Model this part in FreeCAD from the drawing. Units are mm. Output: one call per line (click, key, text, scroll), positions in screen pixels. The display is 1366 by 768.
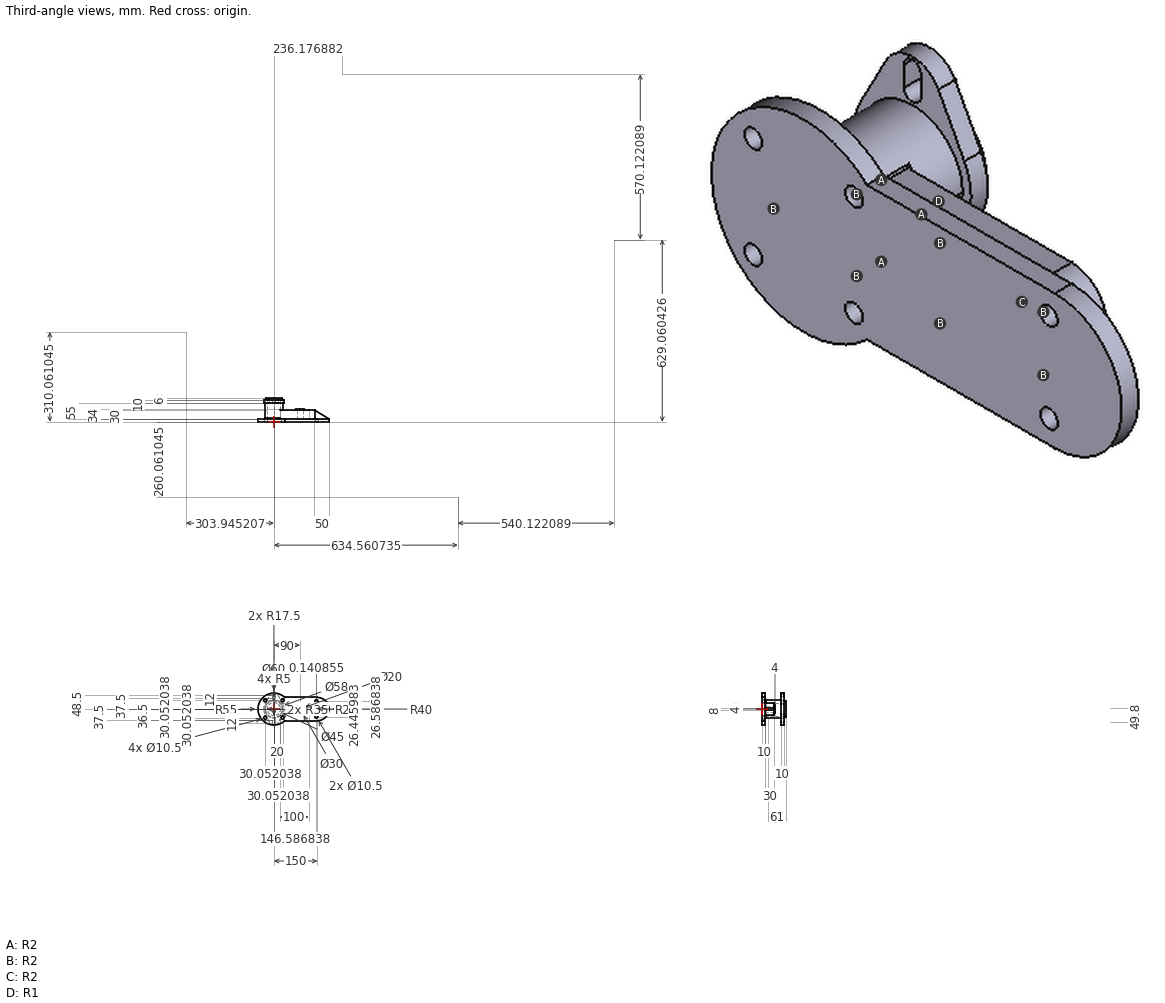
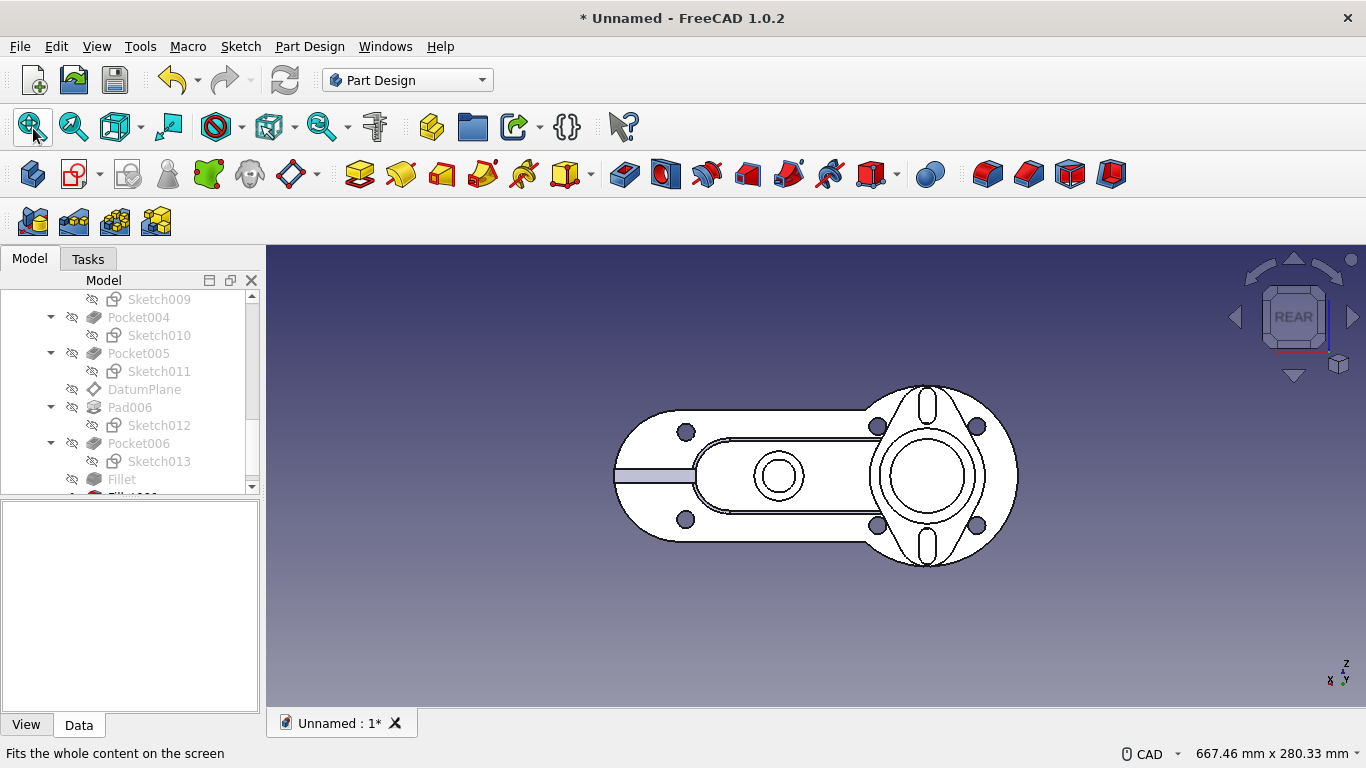
key(v)
key(f)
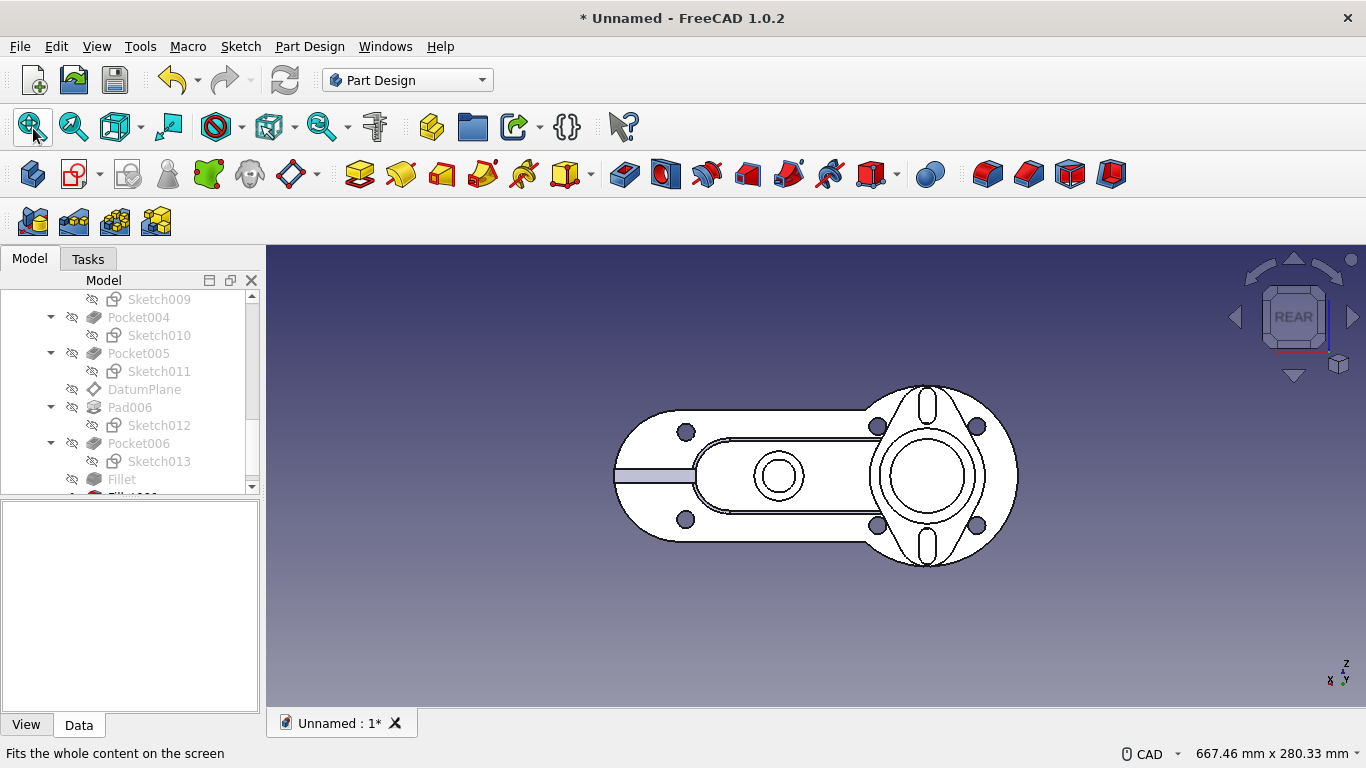
key(6)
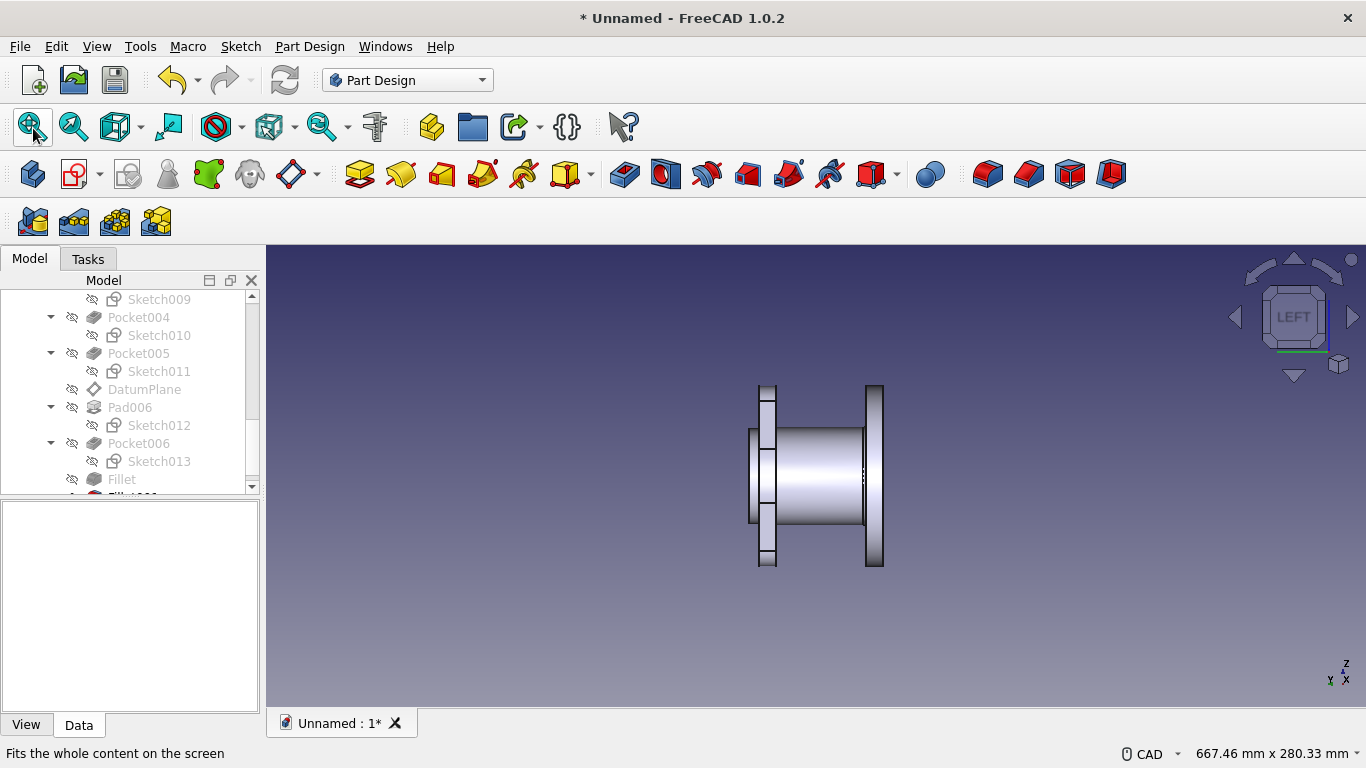
key(v)
key(f)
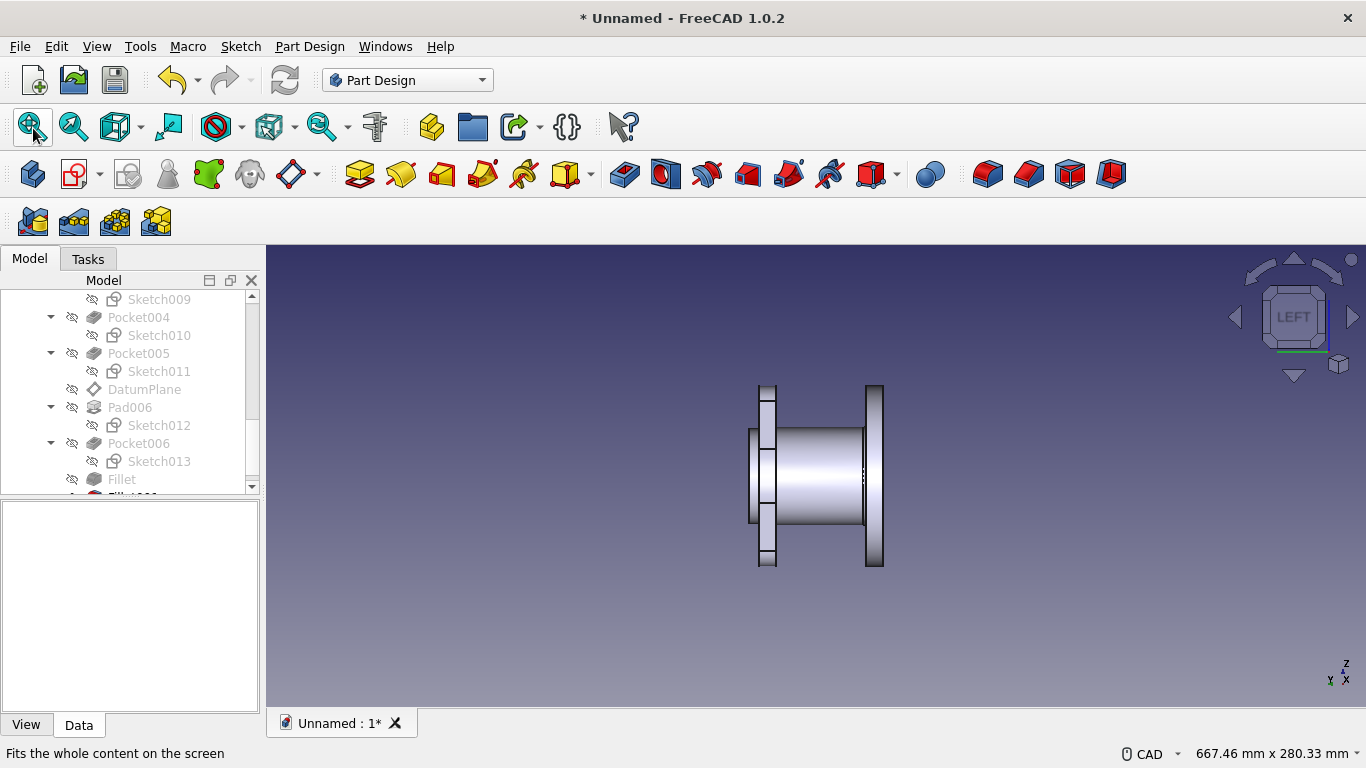
key(v)
key(3)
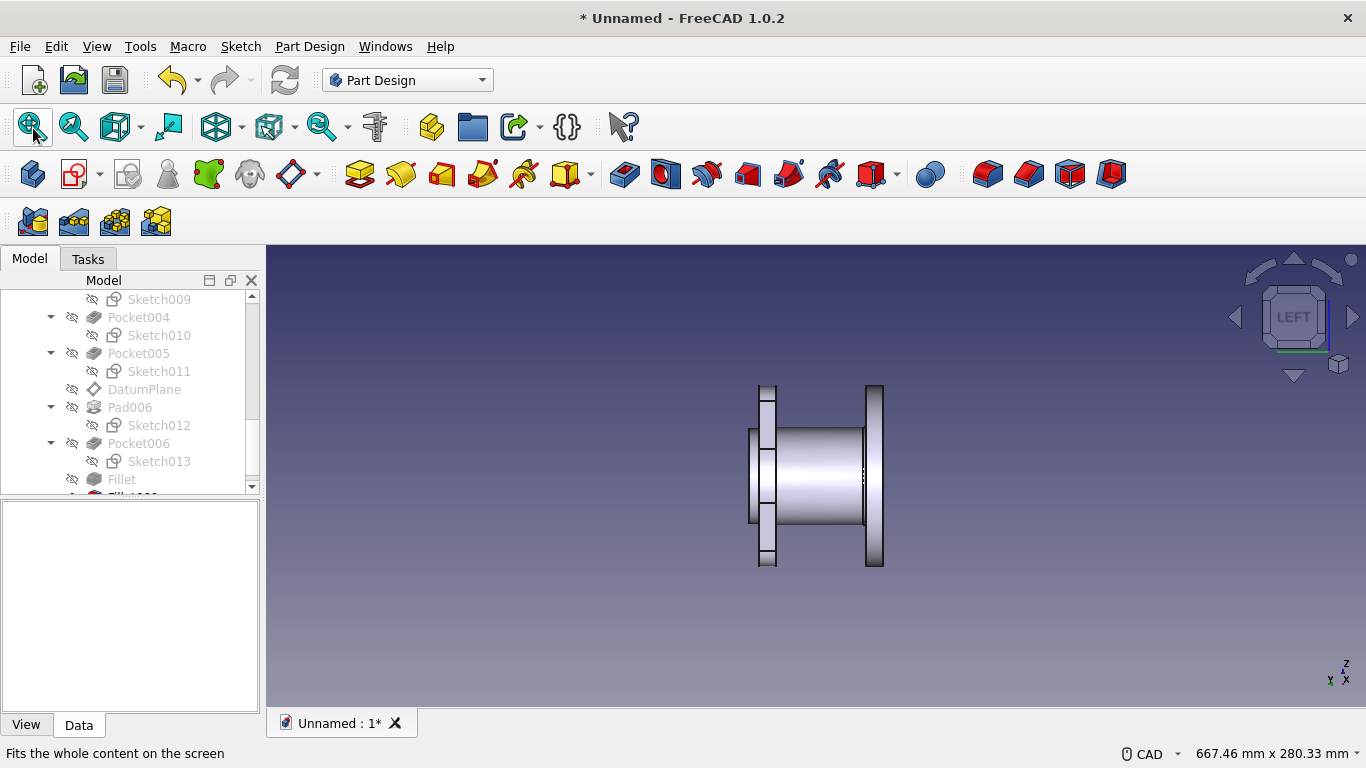
key(0)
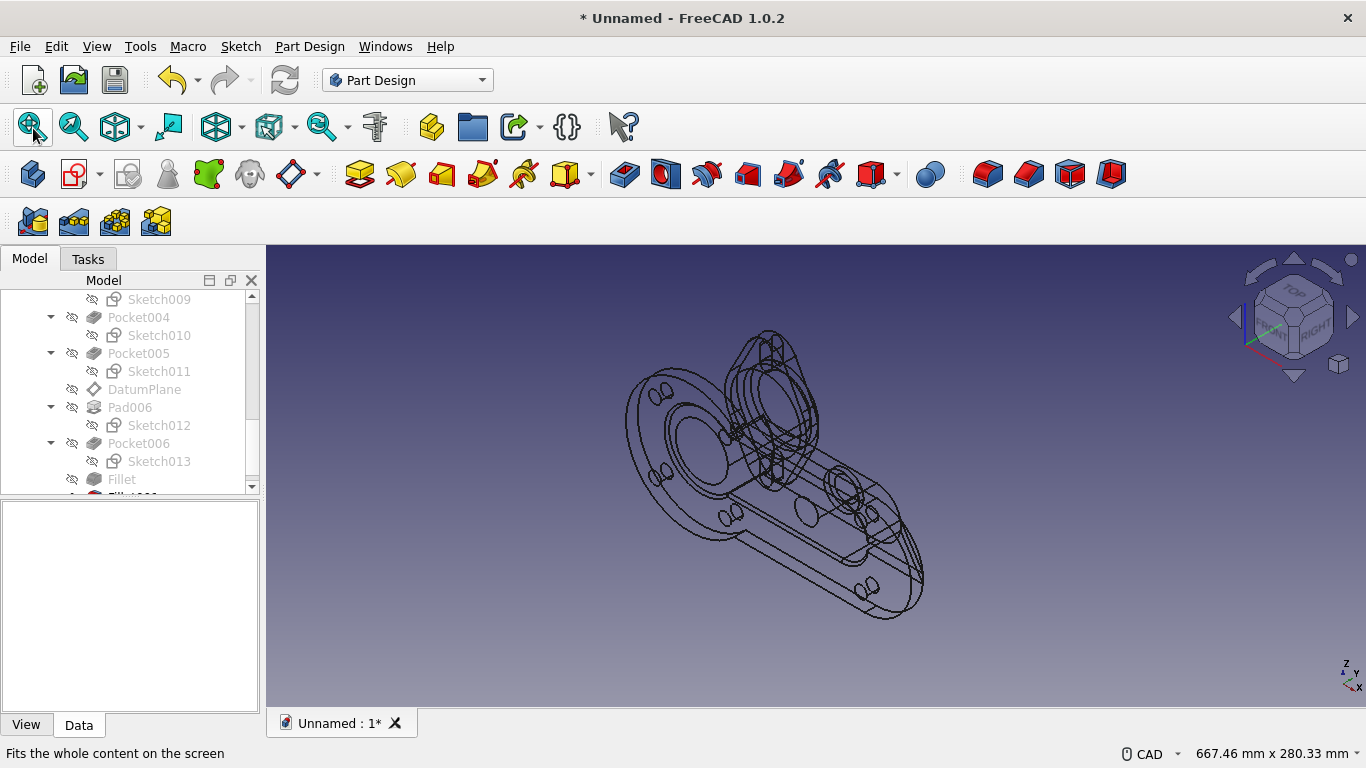
click(847, 513)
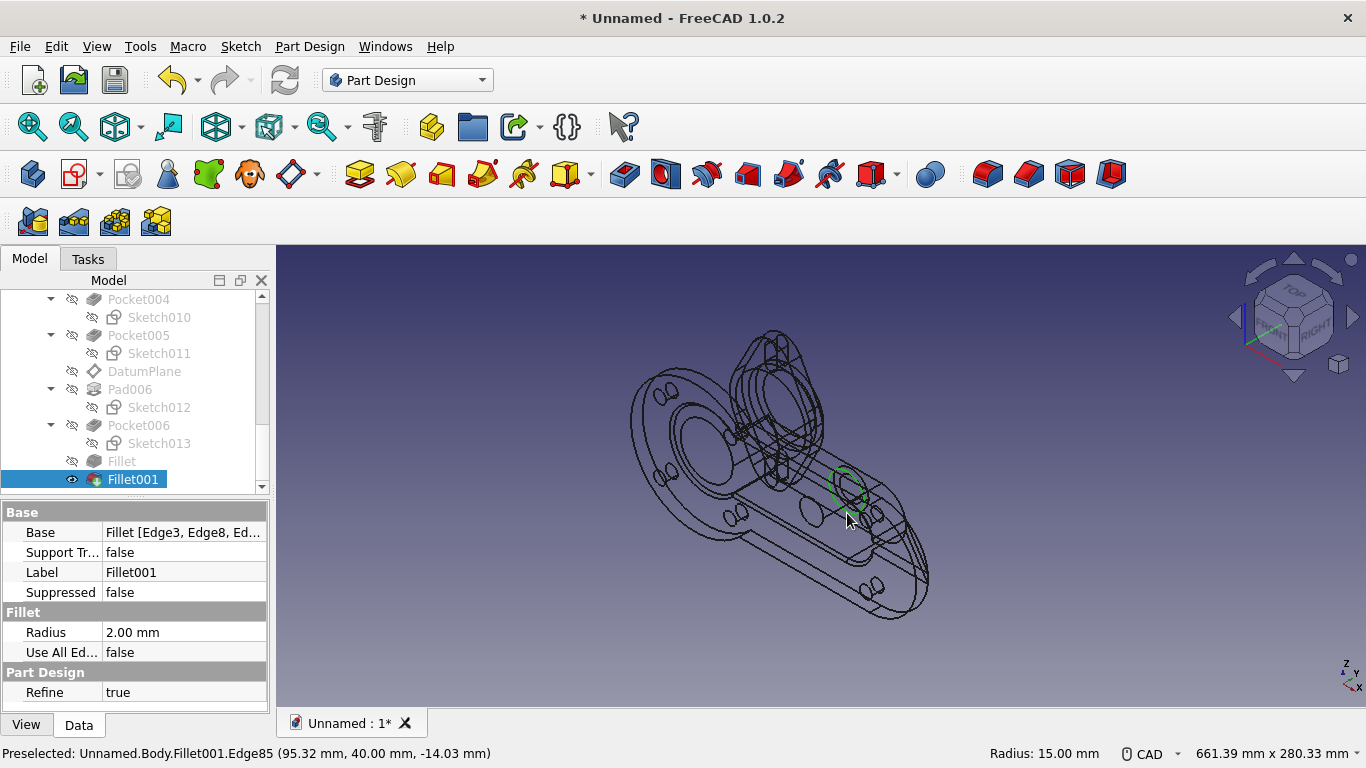
key(v)
key(1)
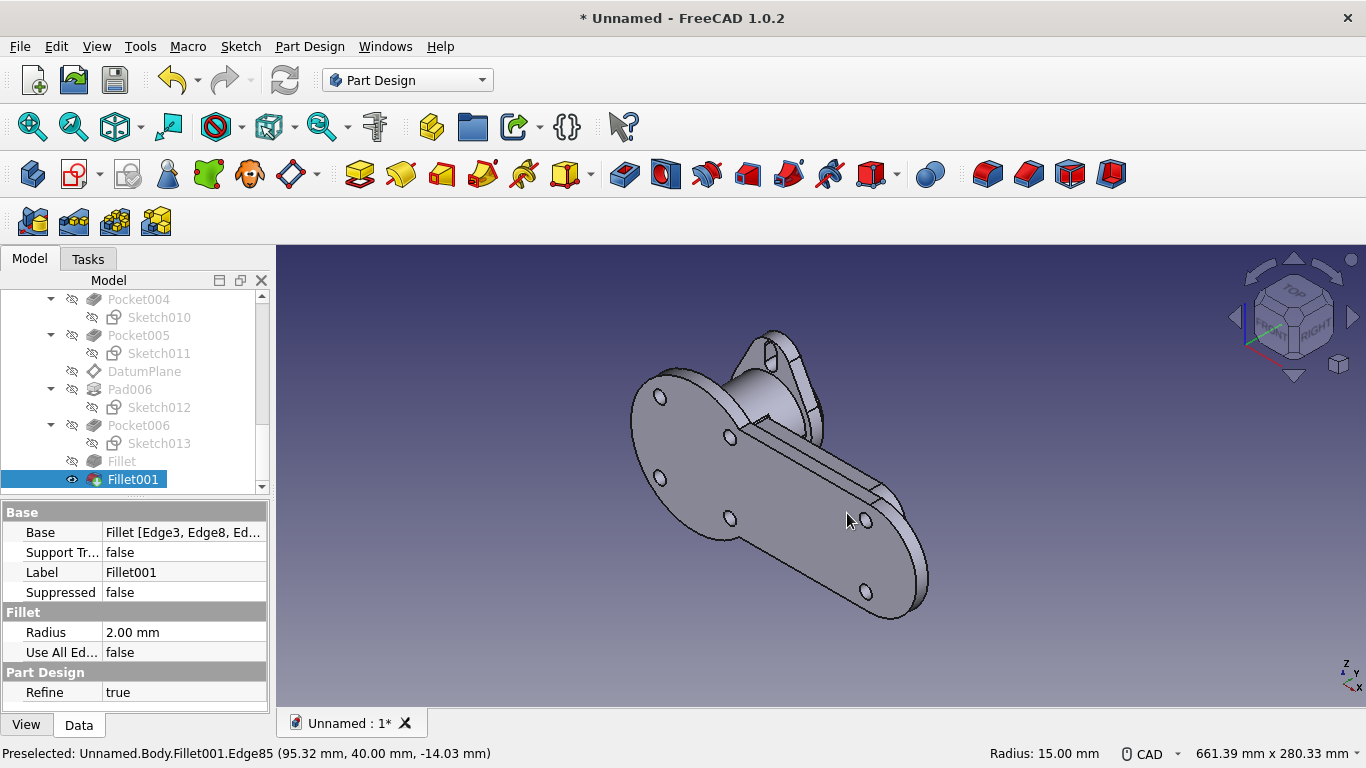
click(988, 174)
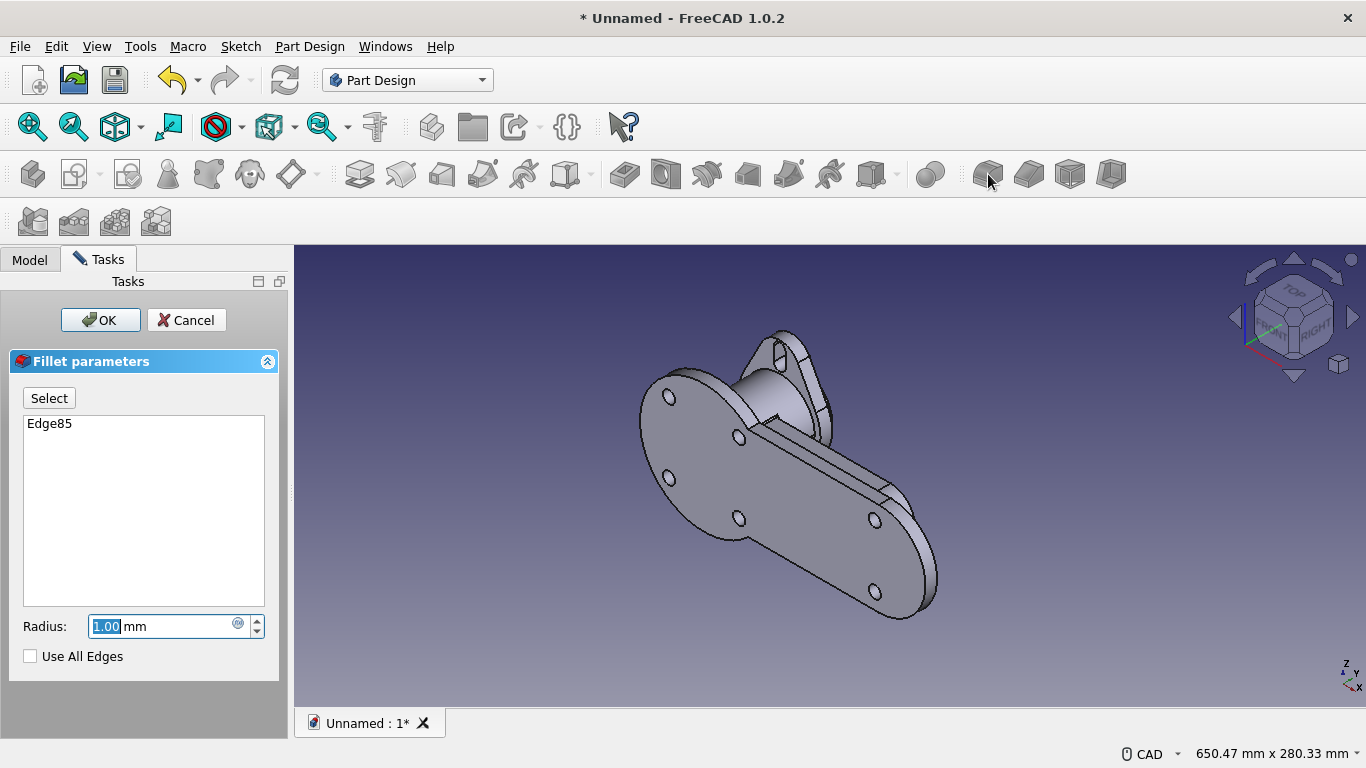
text(2)
key(Tab)